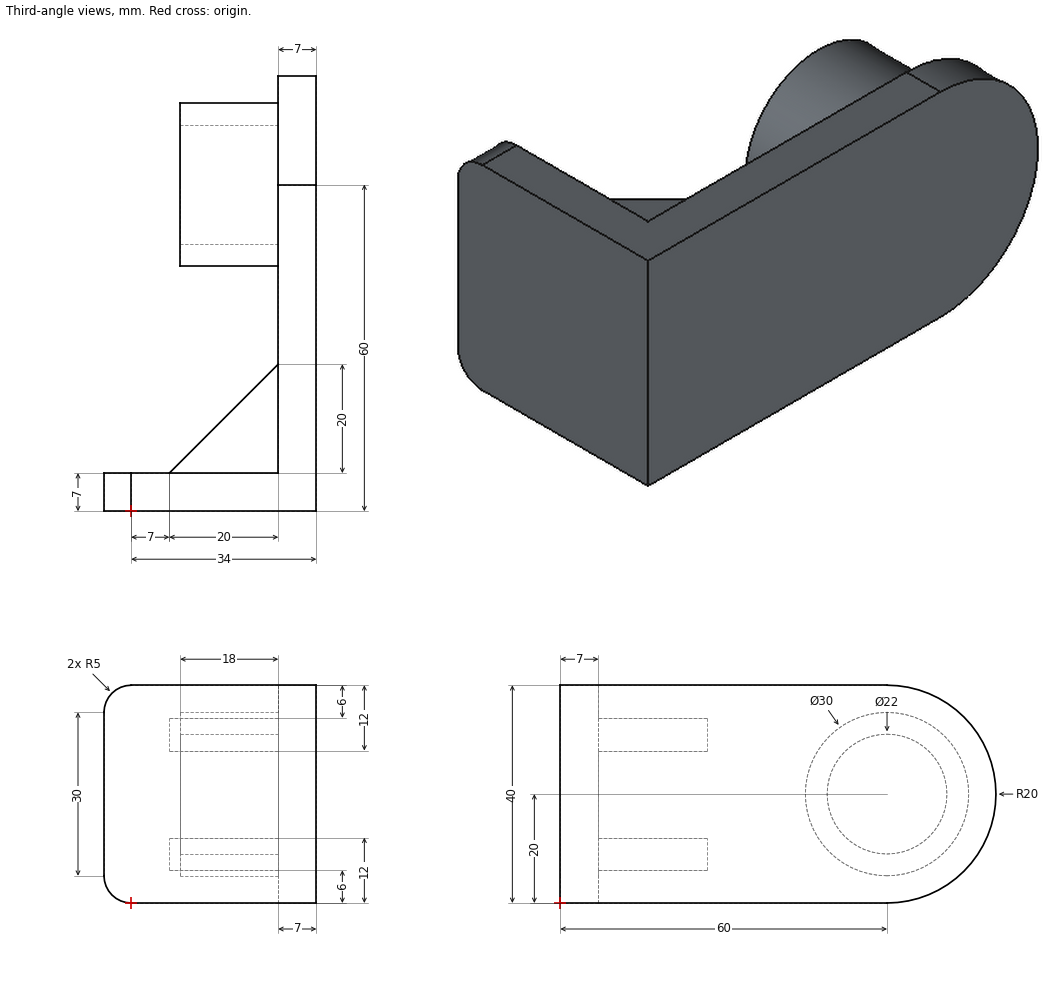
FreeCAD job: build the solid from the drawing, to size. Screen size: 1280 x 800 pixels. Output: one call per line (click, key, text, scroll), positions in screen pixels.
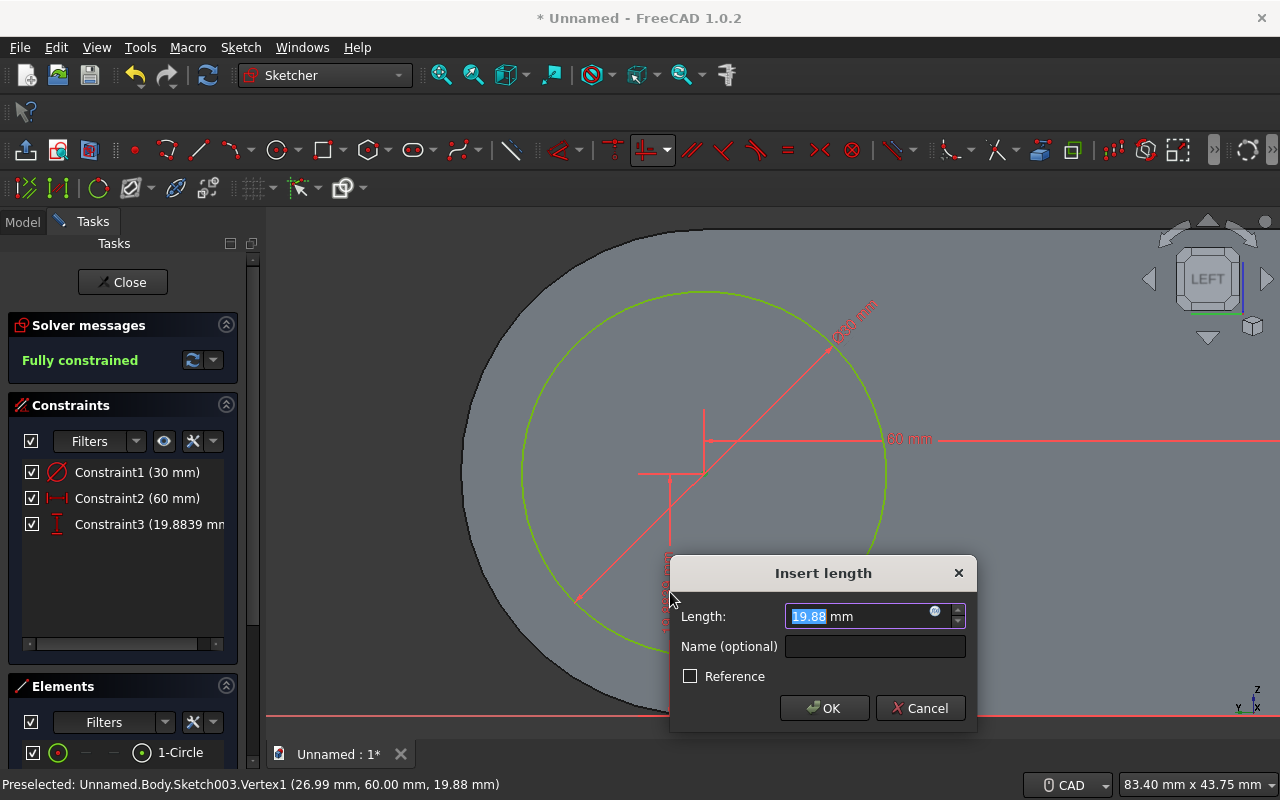
text(20)
key(Return)
key(Escape)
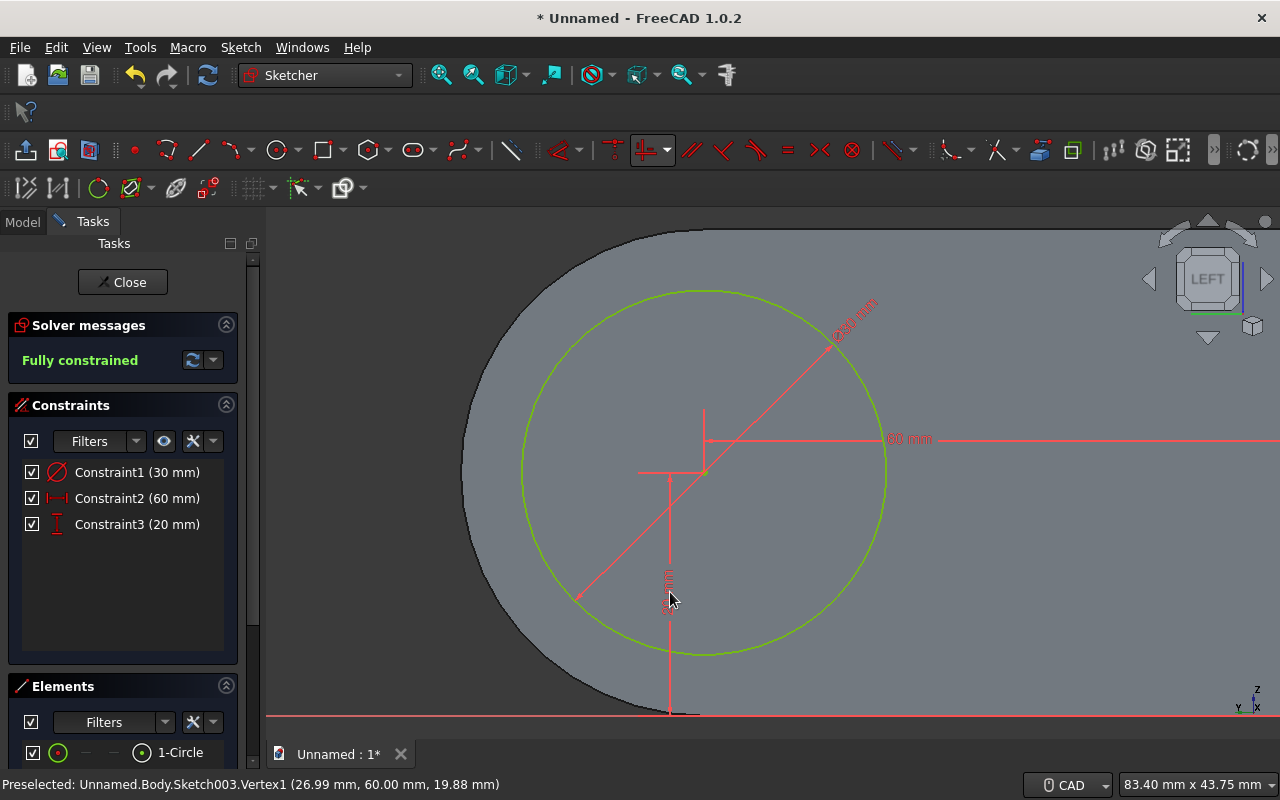
click(123, 282)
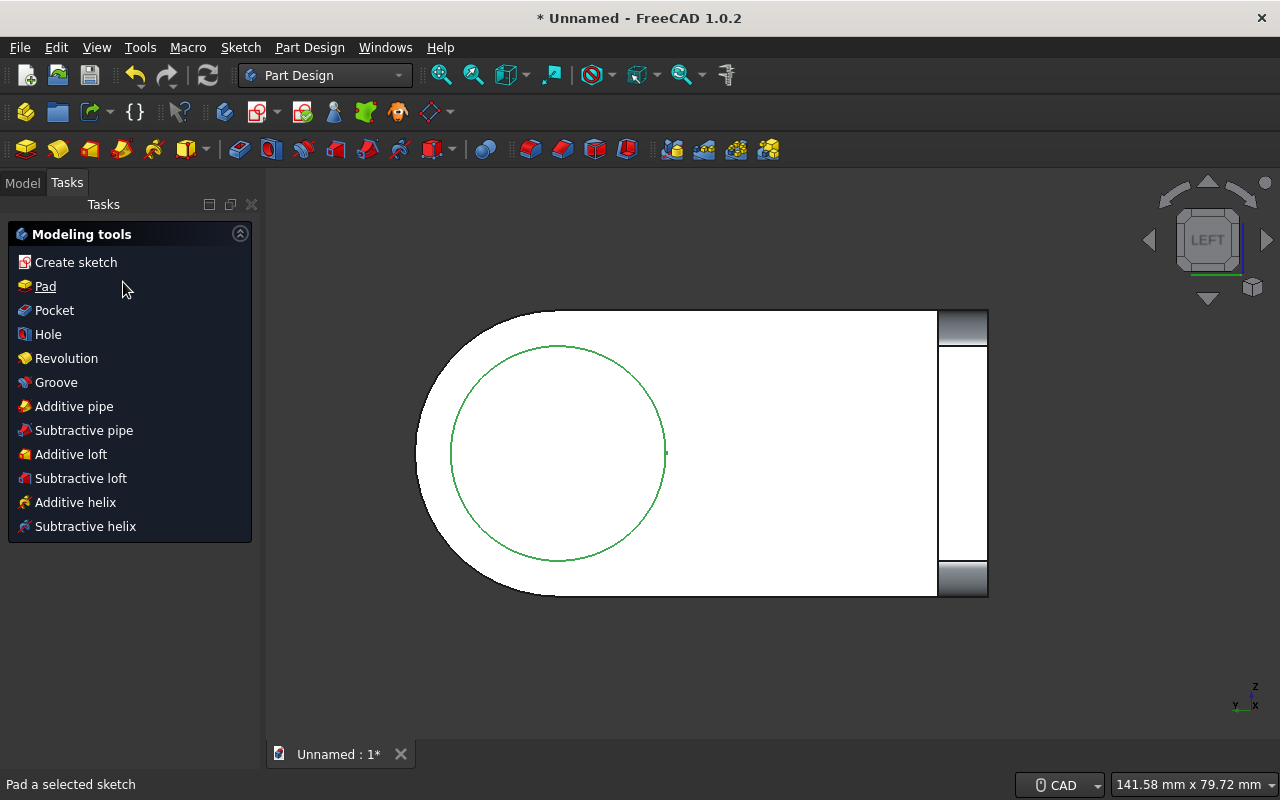
click(26, 150)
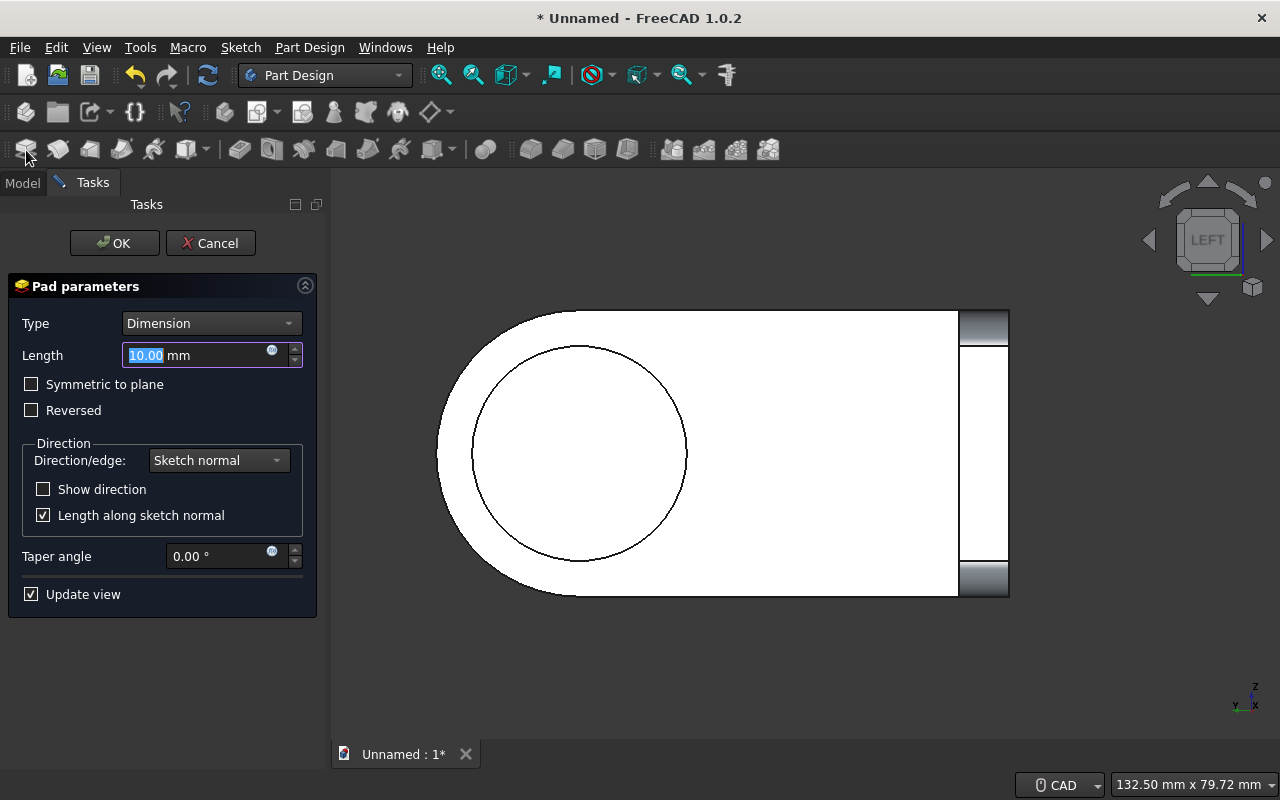
text(18)
key(Tab)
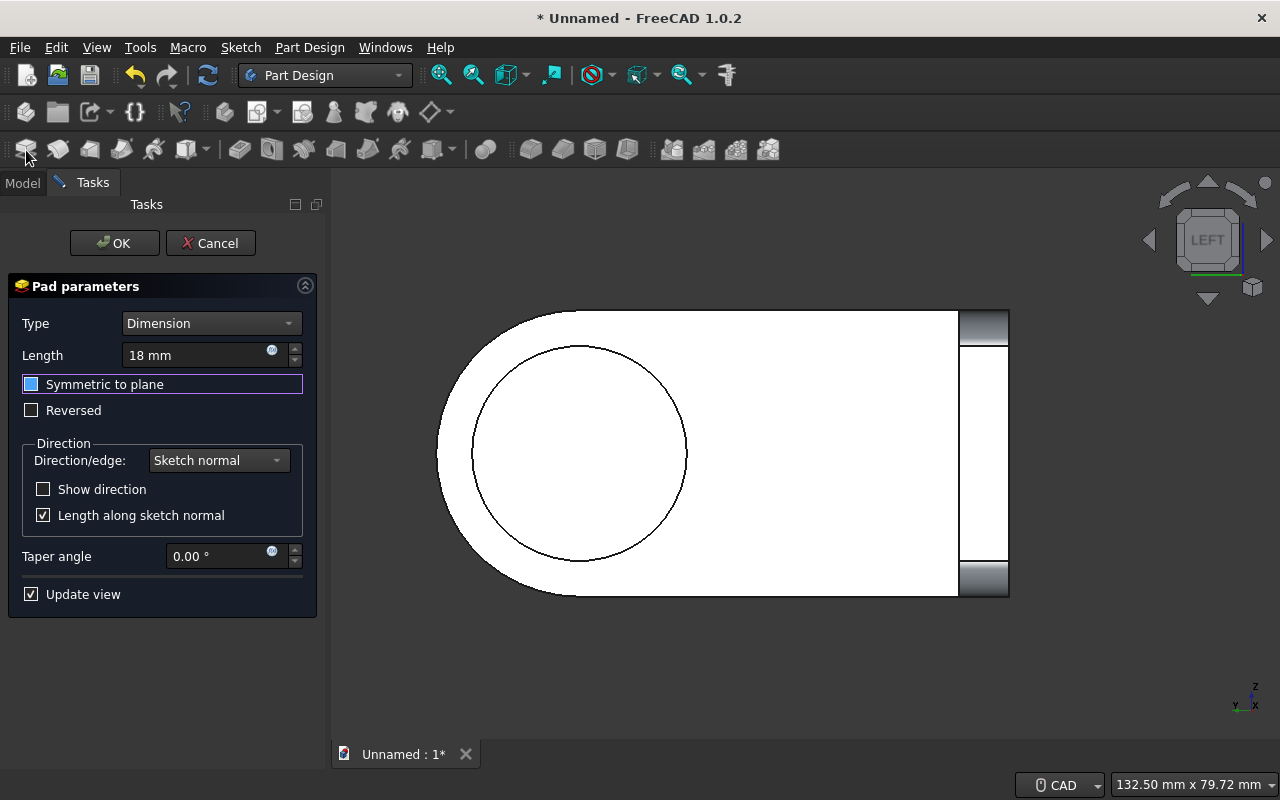
click(115, 243)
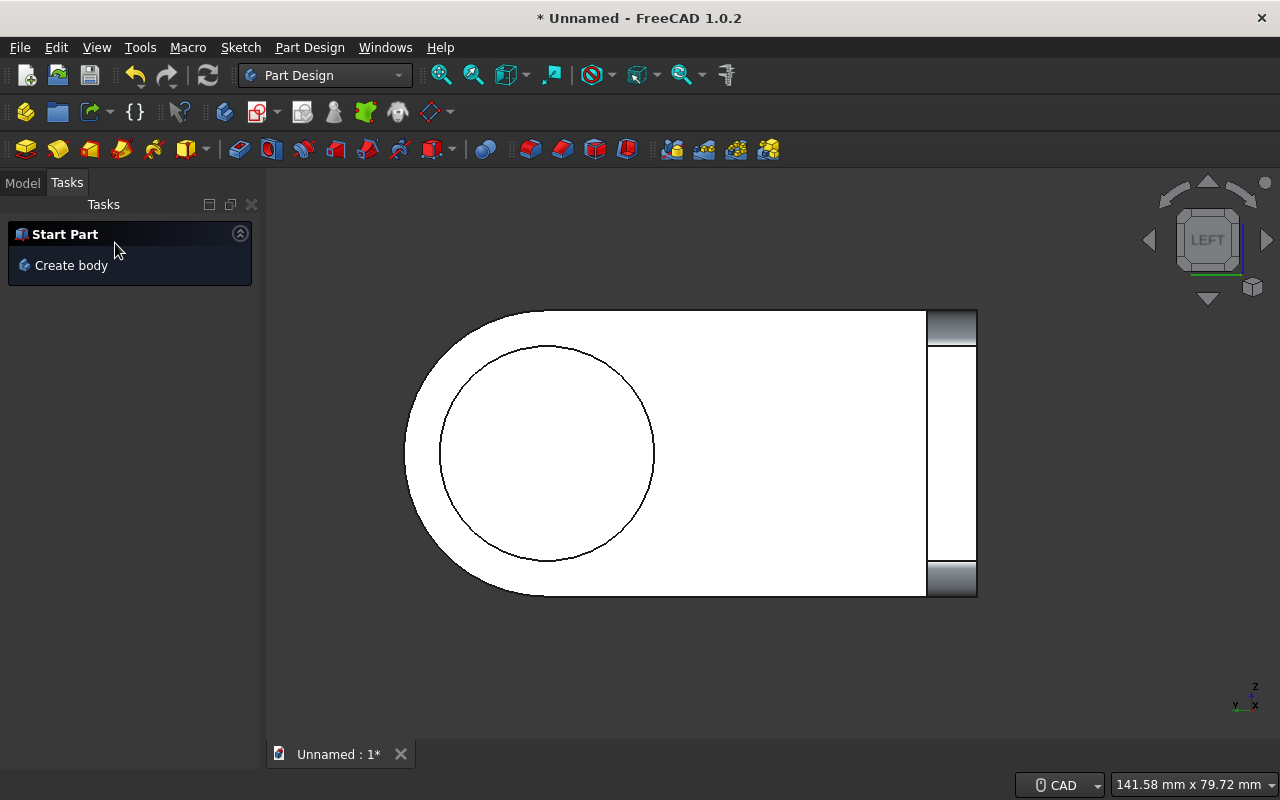
click(547, 453)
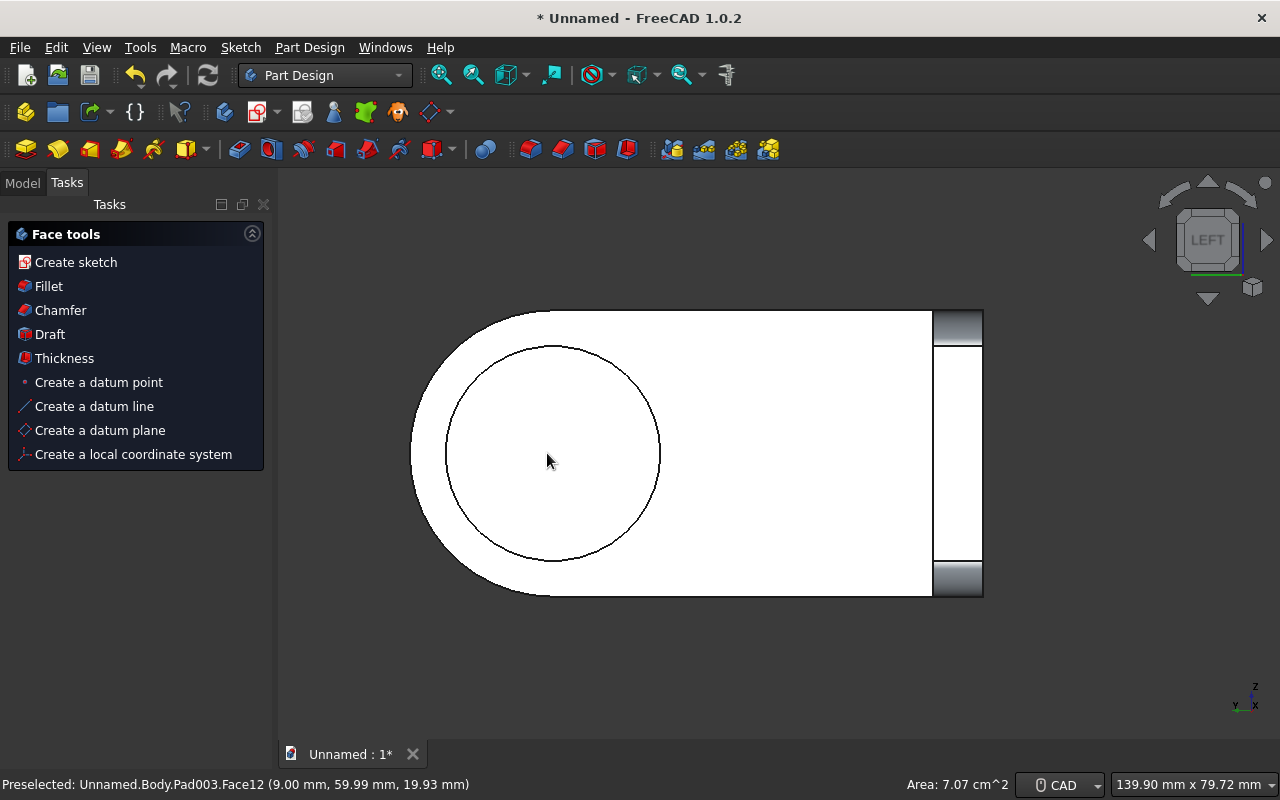
click(258, 112)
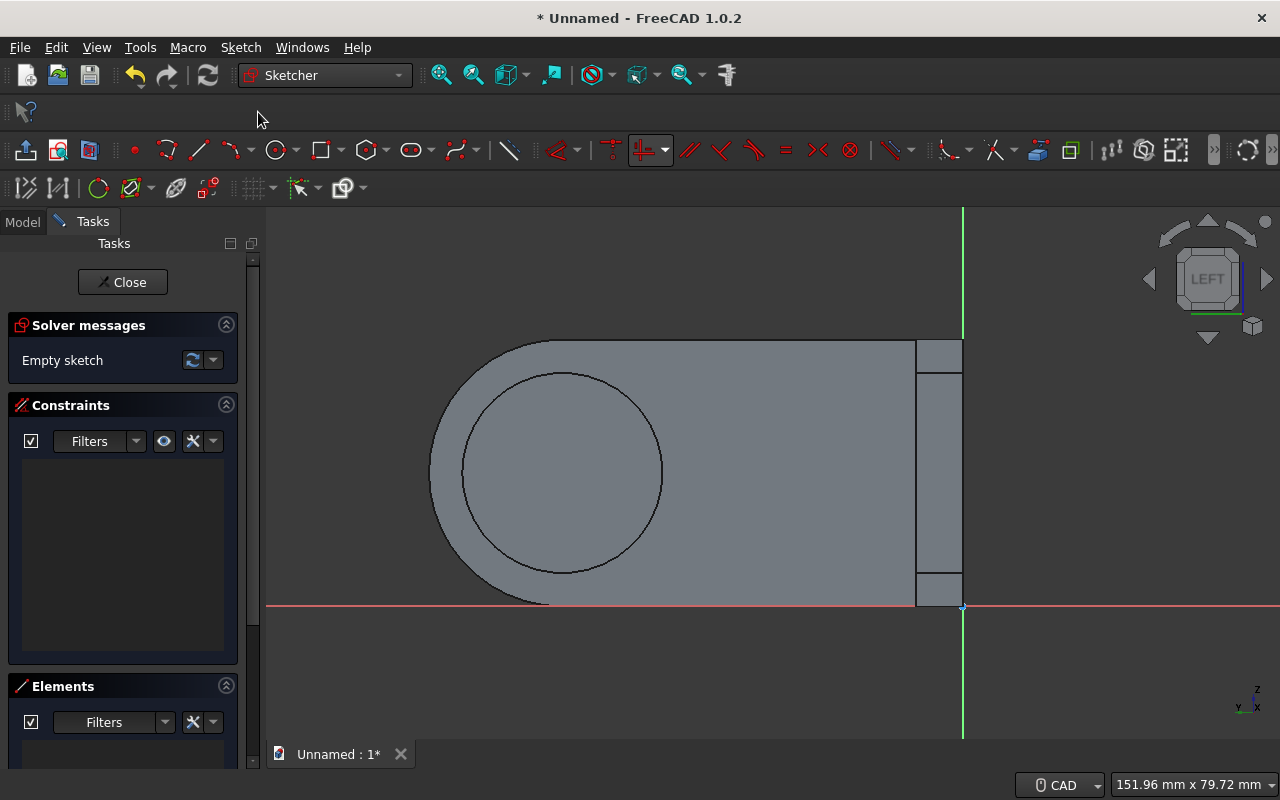
click(90, 150)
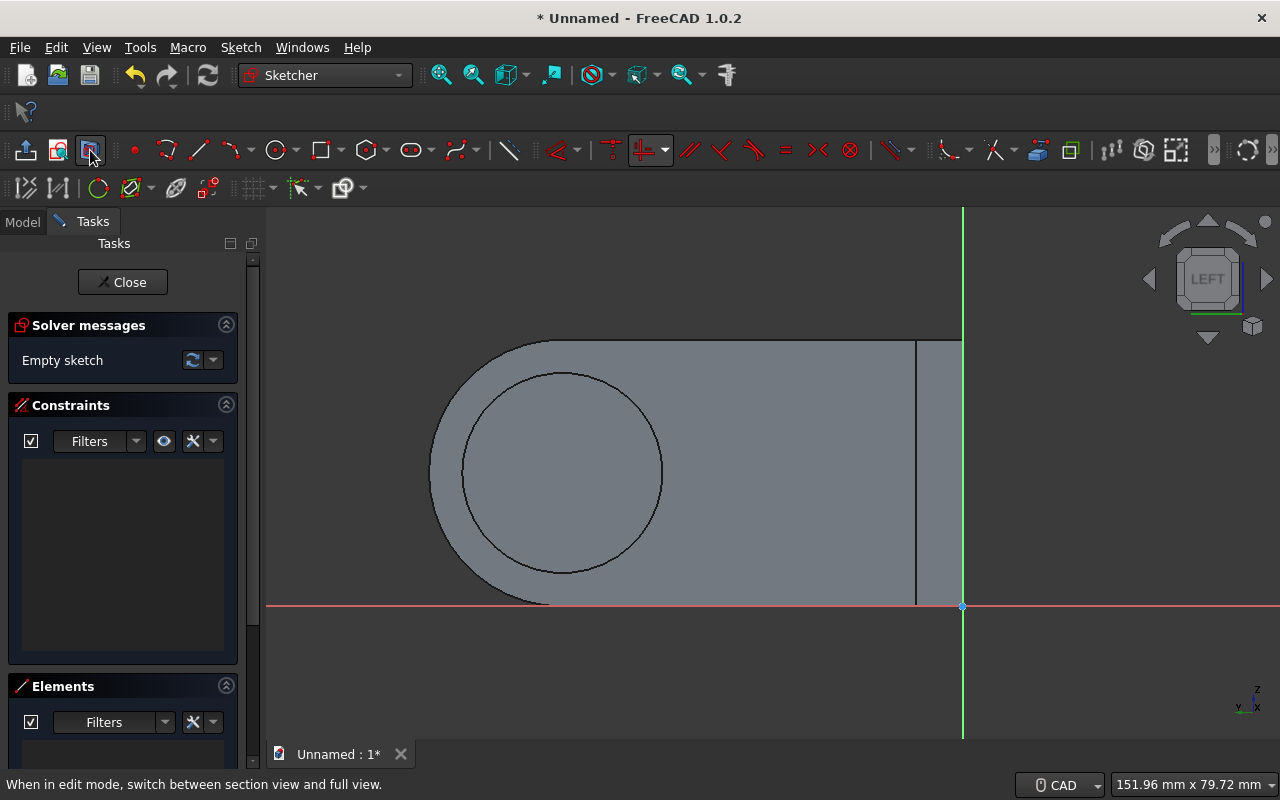
scroll(446, 473, up, 4)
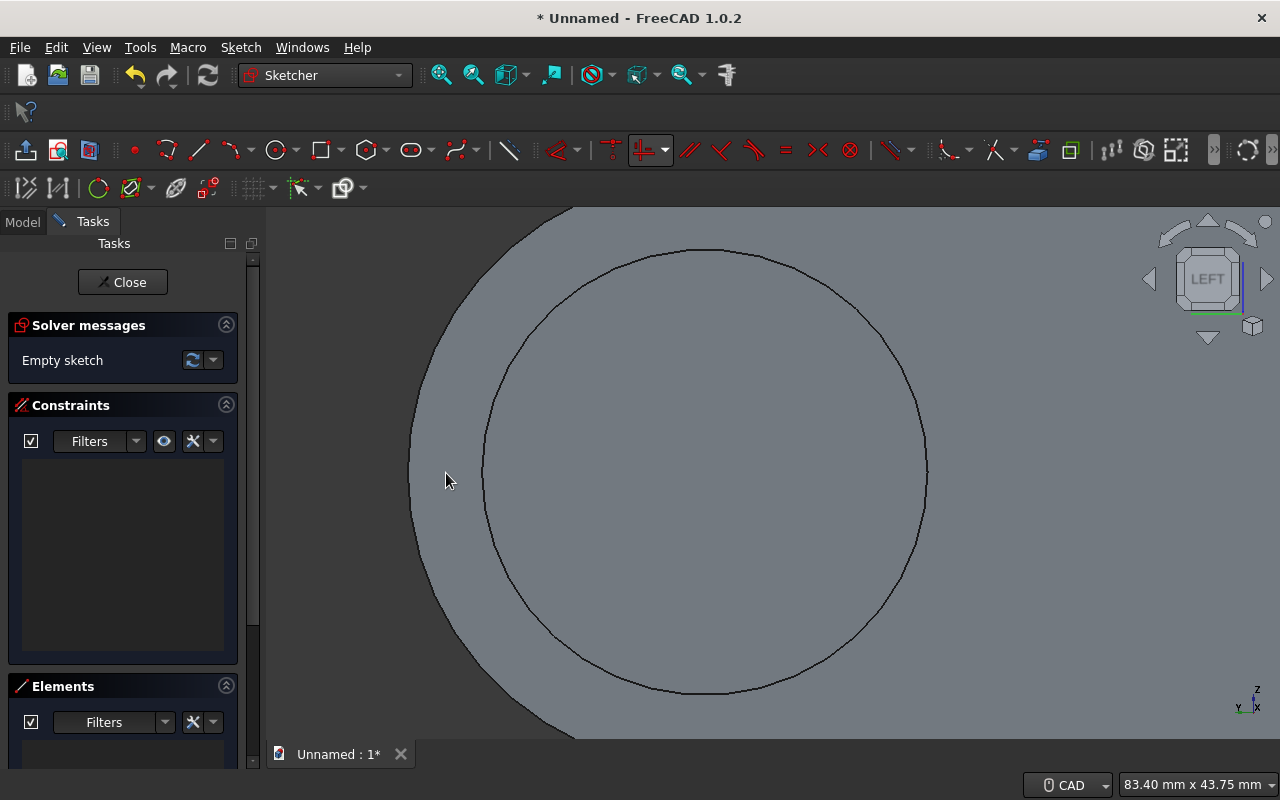
click(276, 150)